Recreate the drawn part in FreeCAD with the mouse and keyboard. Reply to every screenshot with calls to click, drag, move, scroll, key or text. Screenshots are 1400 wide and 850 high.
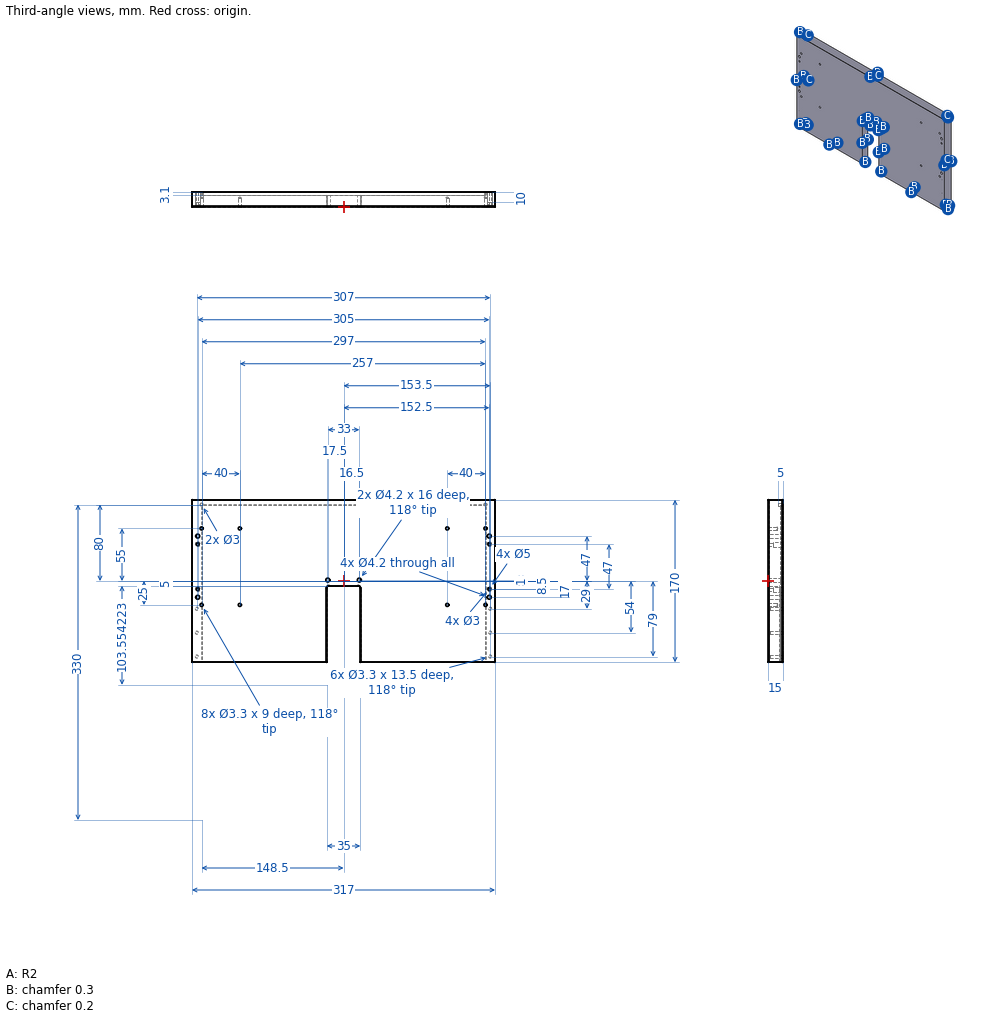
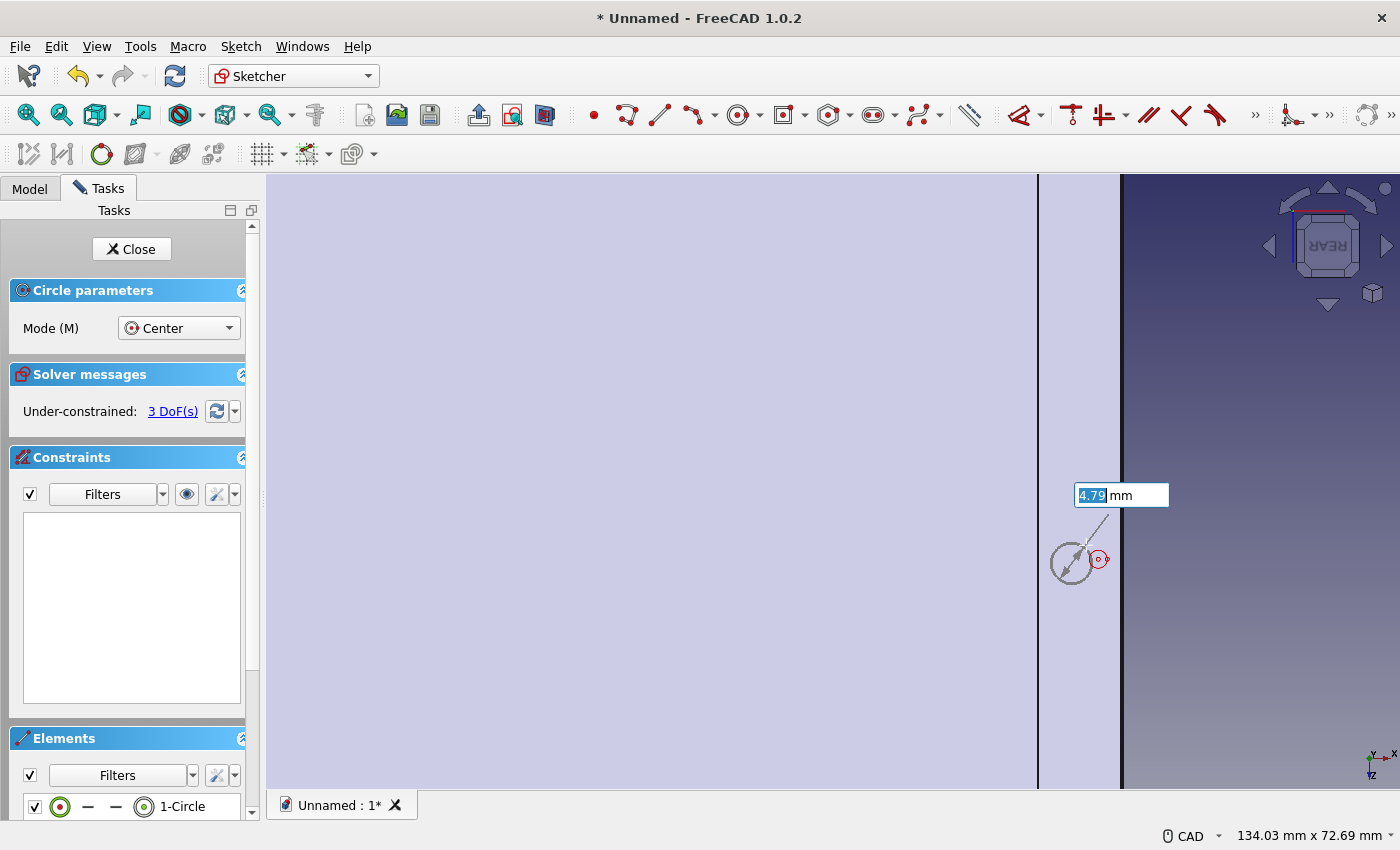
click(1085, 545)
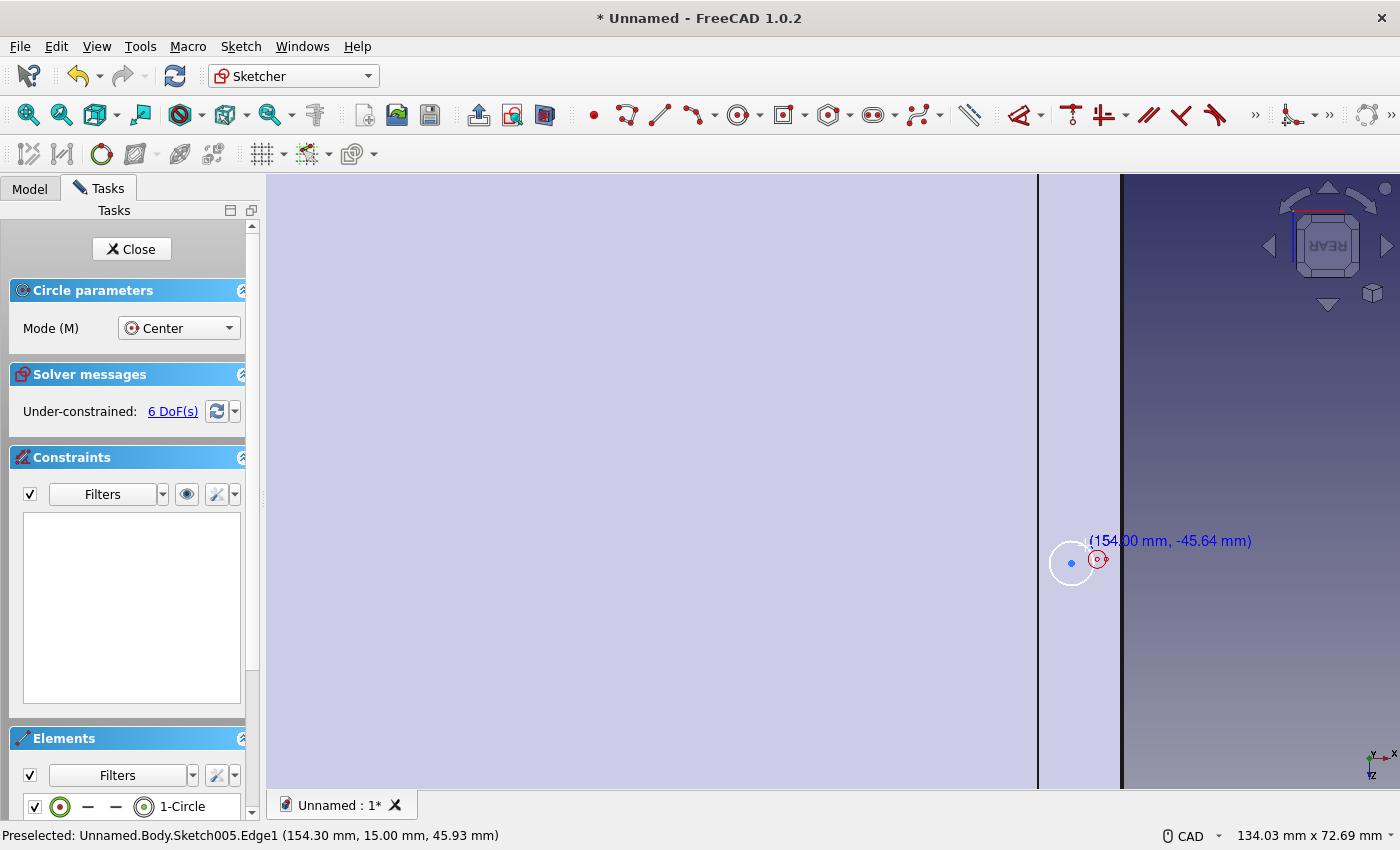
scroll(1086, 545, down, 7)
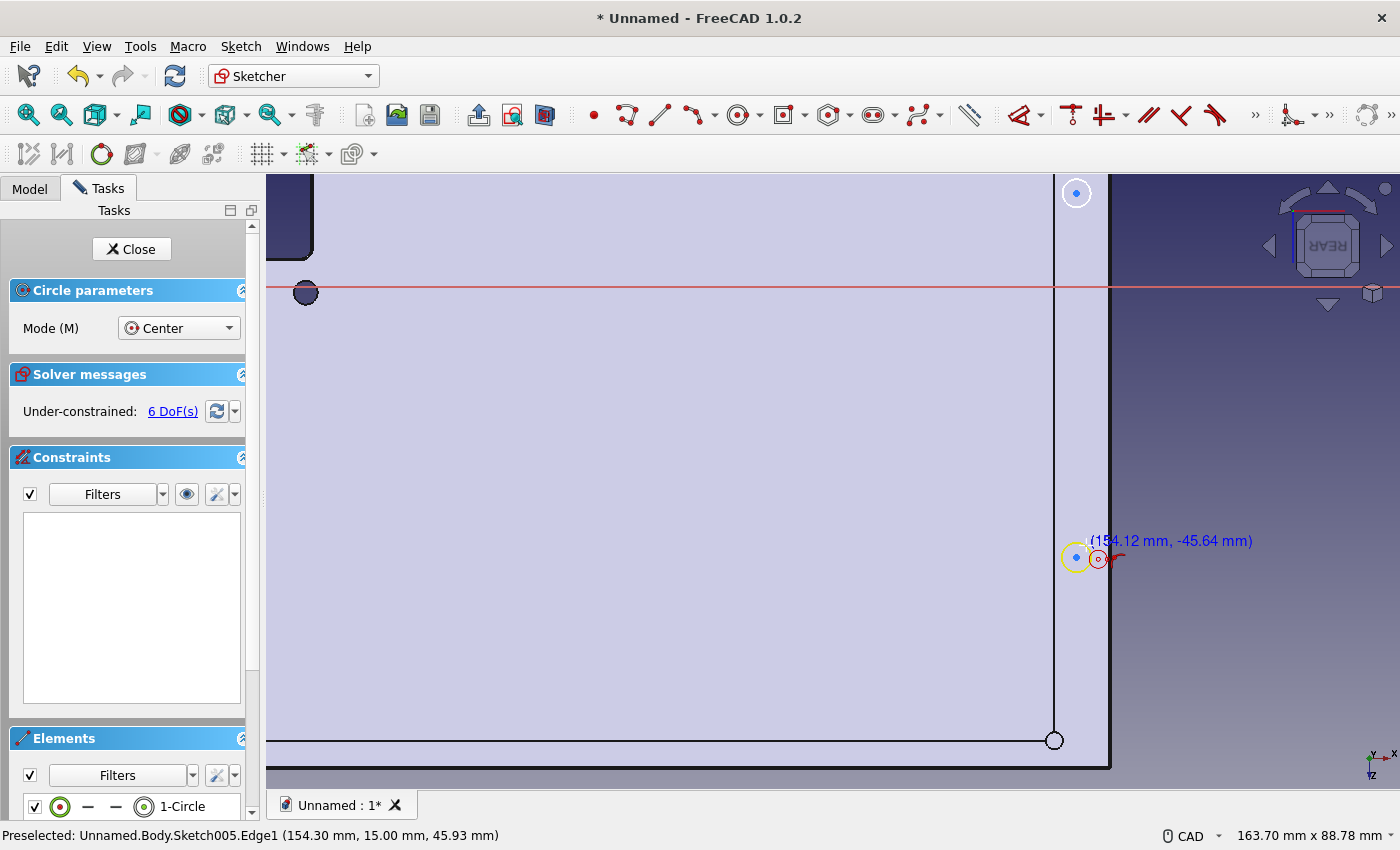
scroll(447, 415, up, 9)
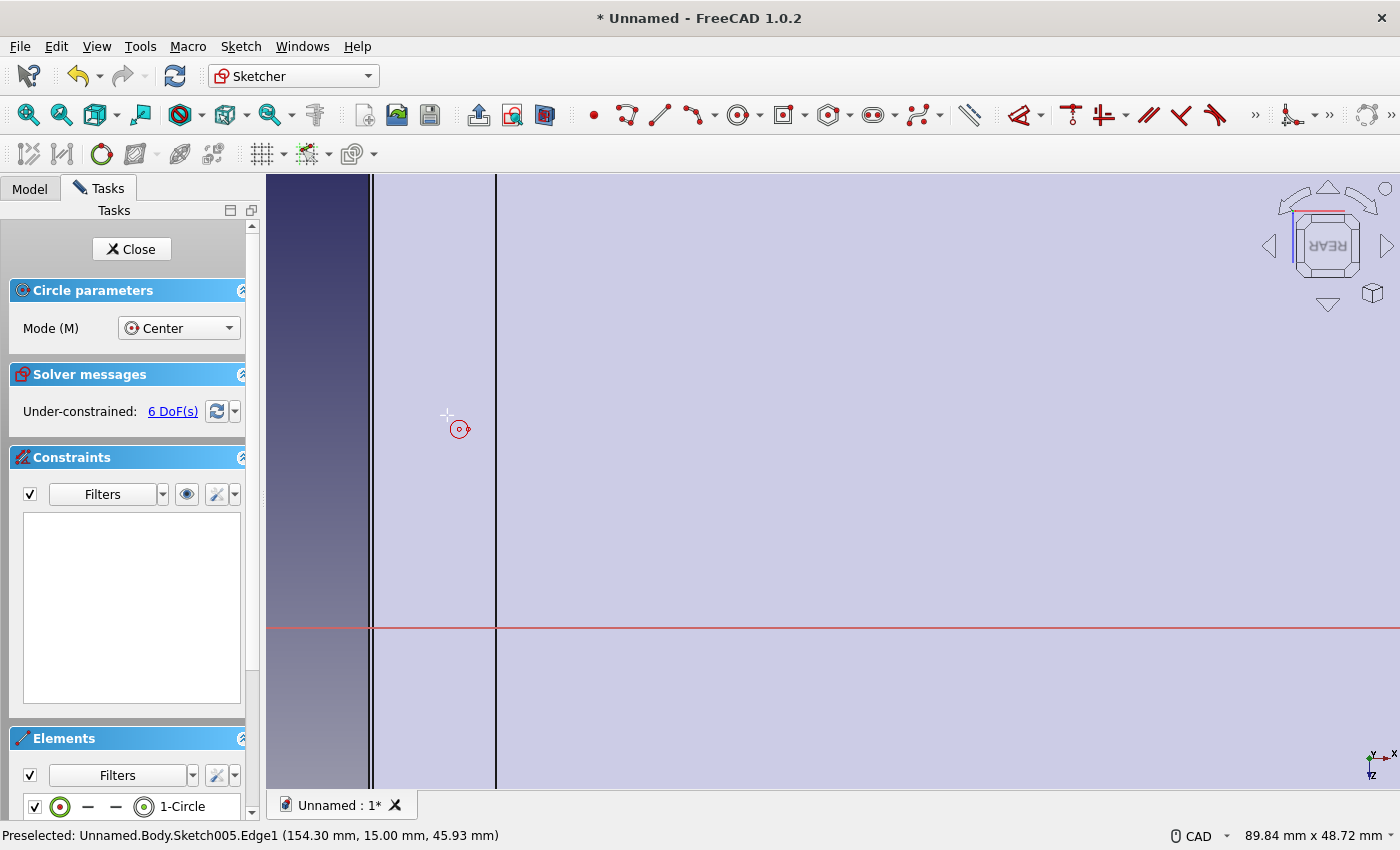
scroll(447, 415, down, 9)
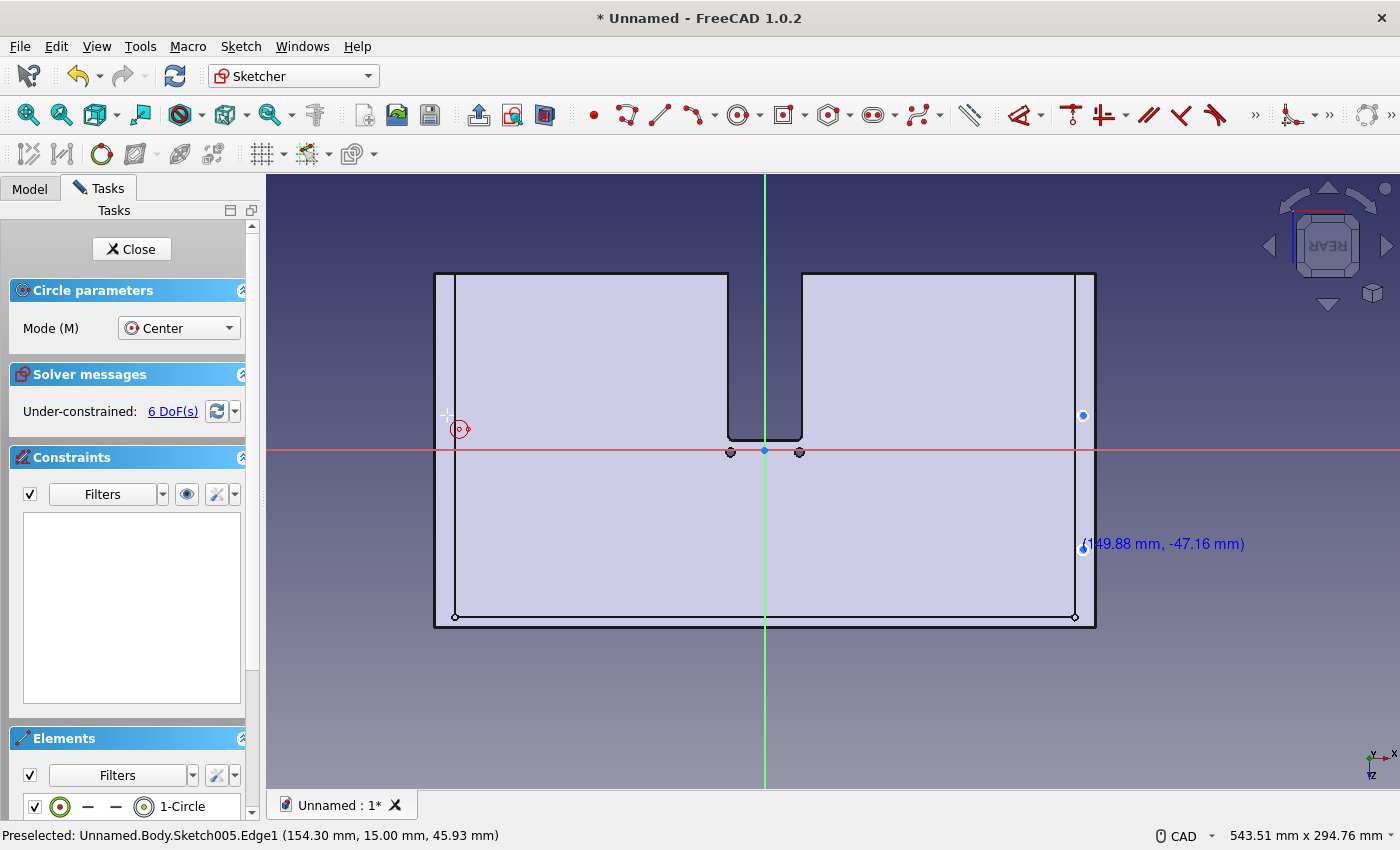
click(447, 415)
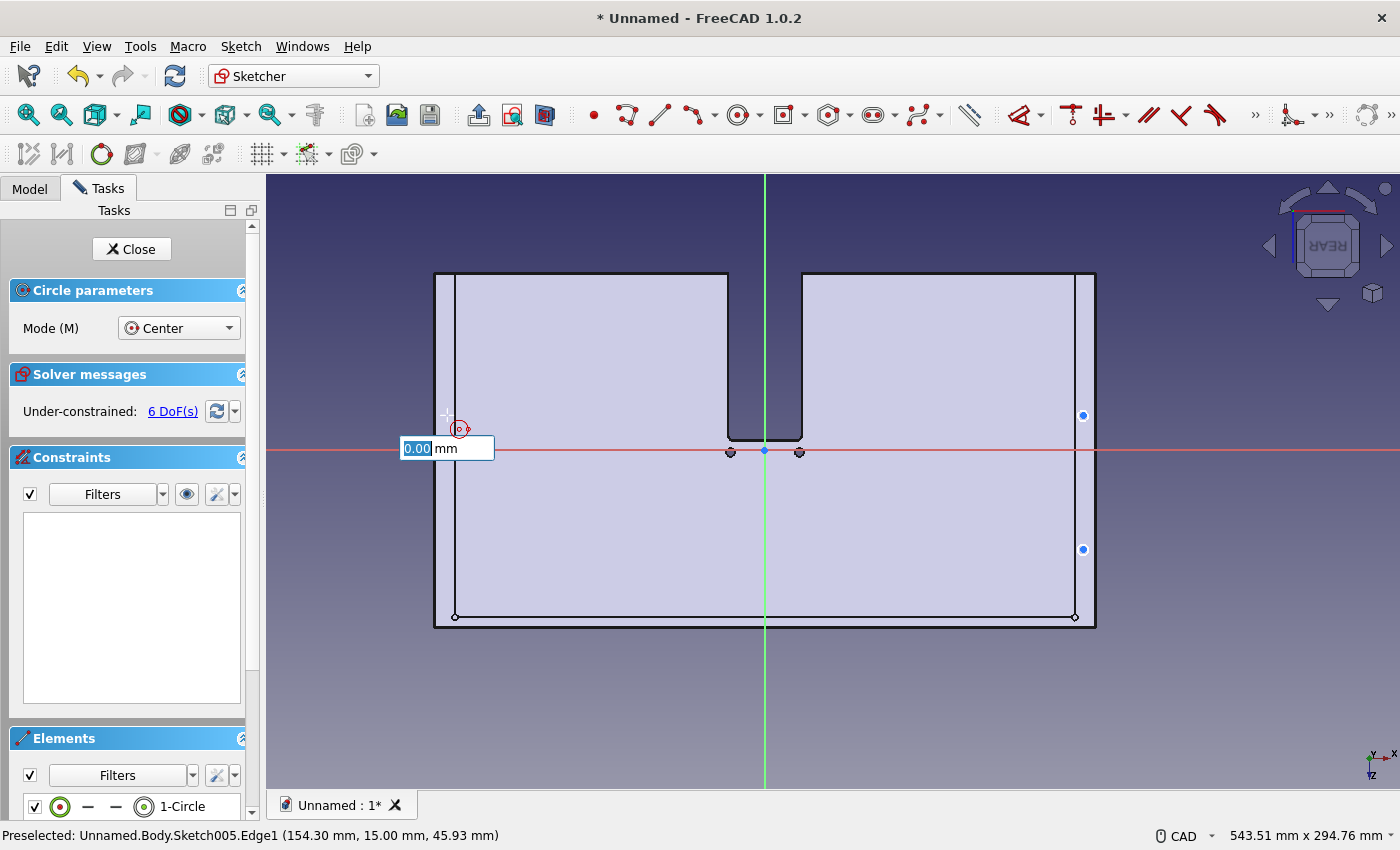
scroll(450, 412, up, 7)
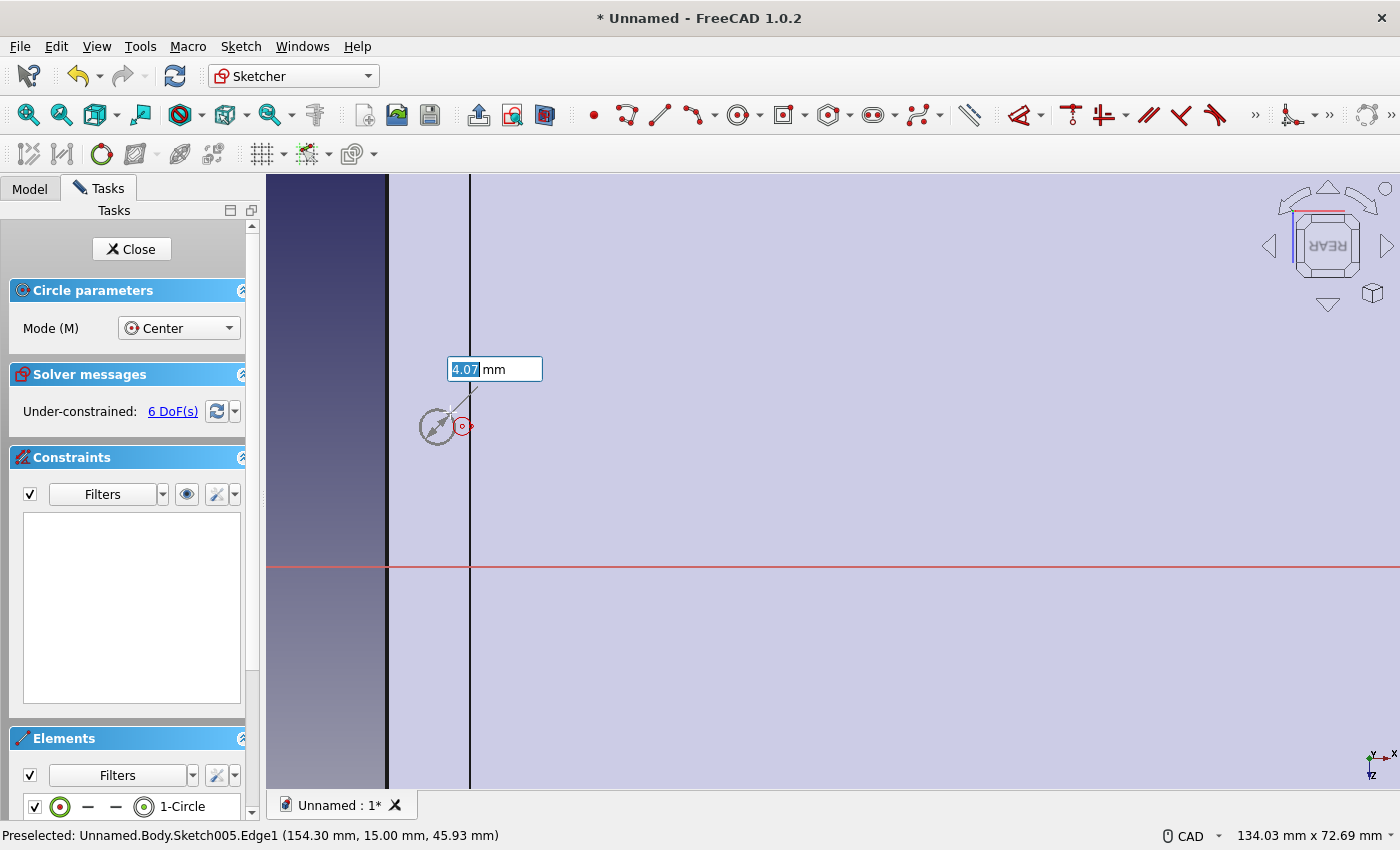
click(449, 410)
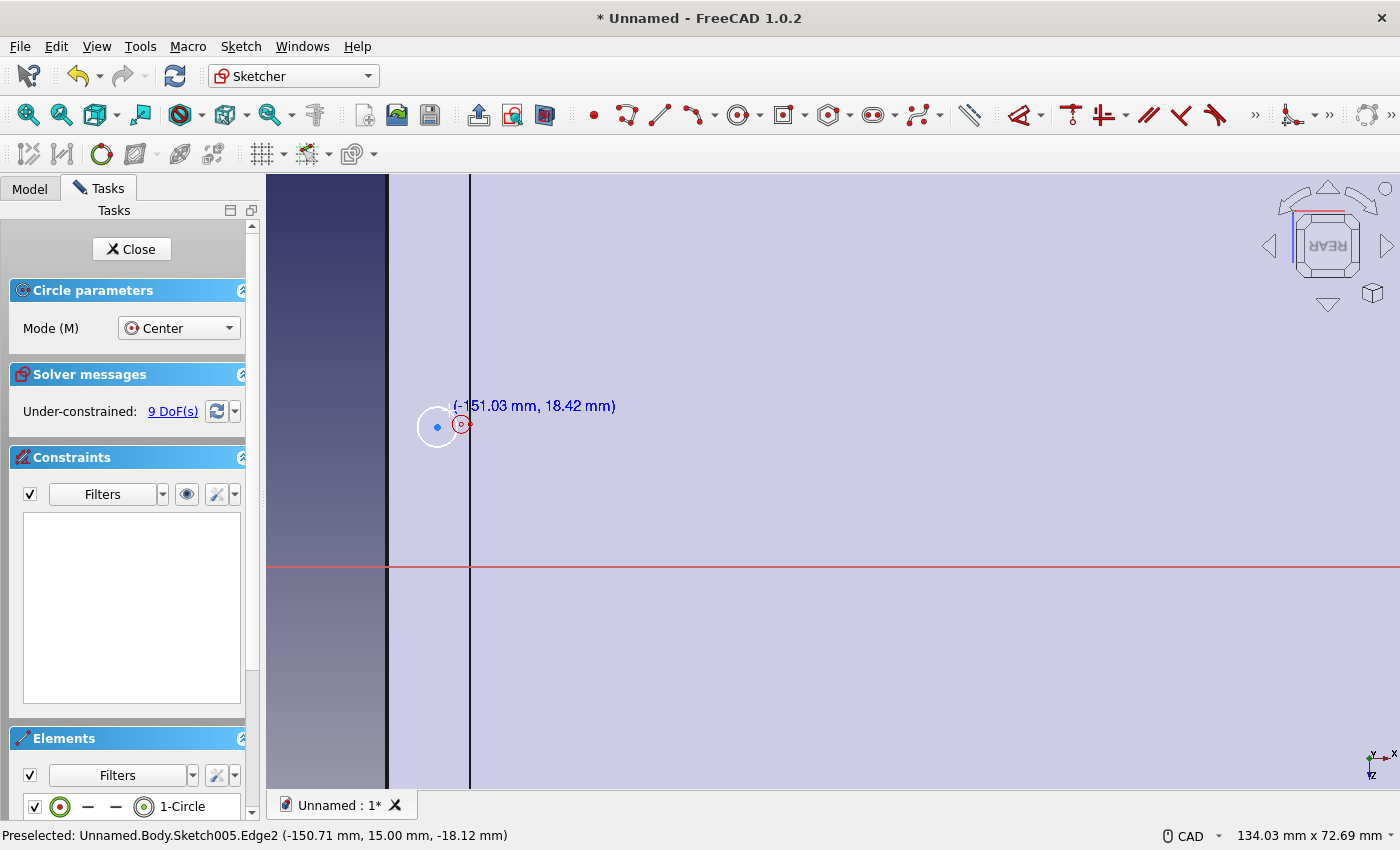
scroll(450, 412, down, 7)